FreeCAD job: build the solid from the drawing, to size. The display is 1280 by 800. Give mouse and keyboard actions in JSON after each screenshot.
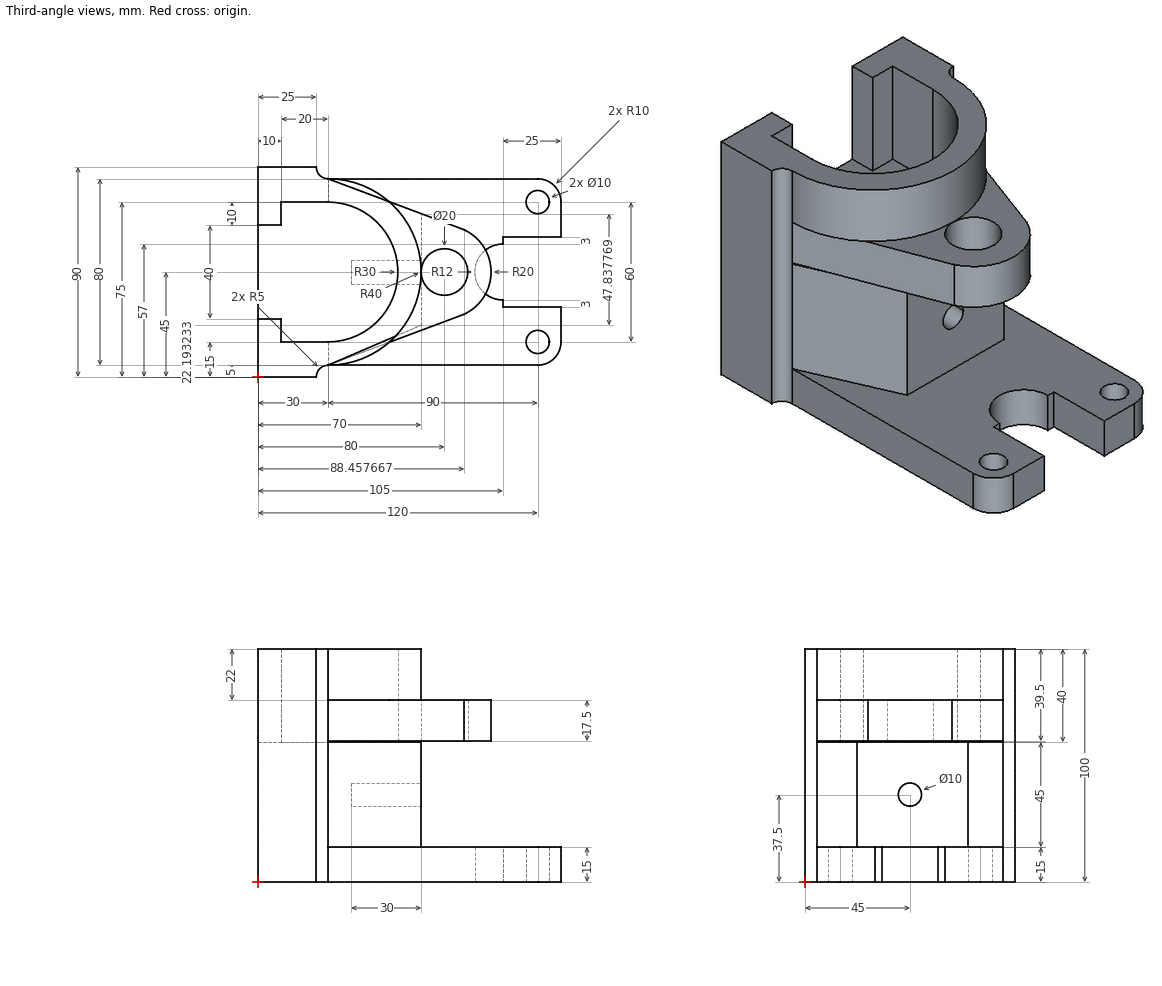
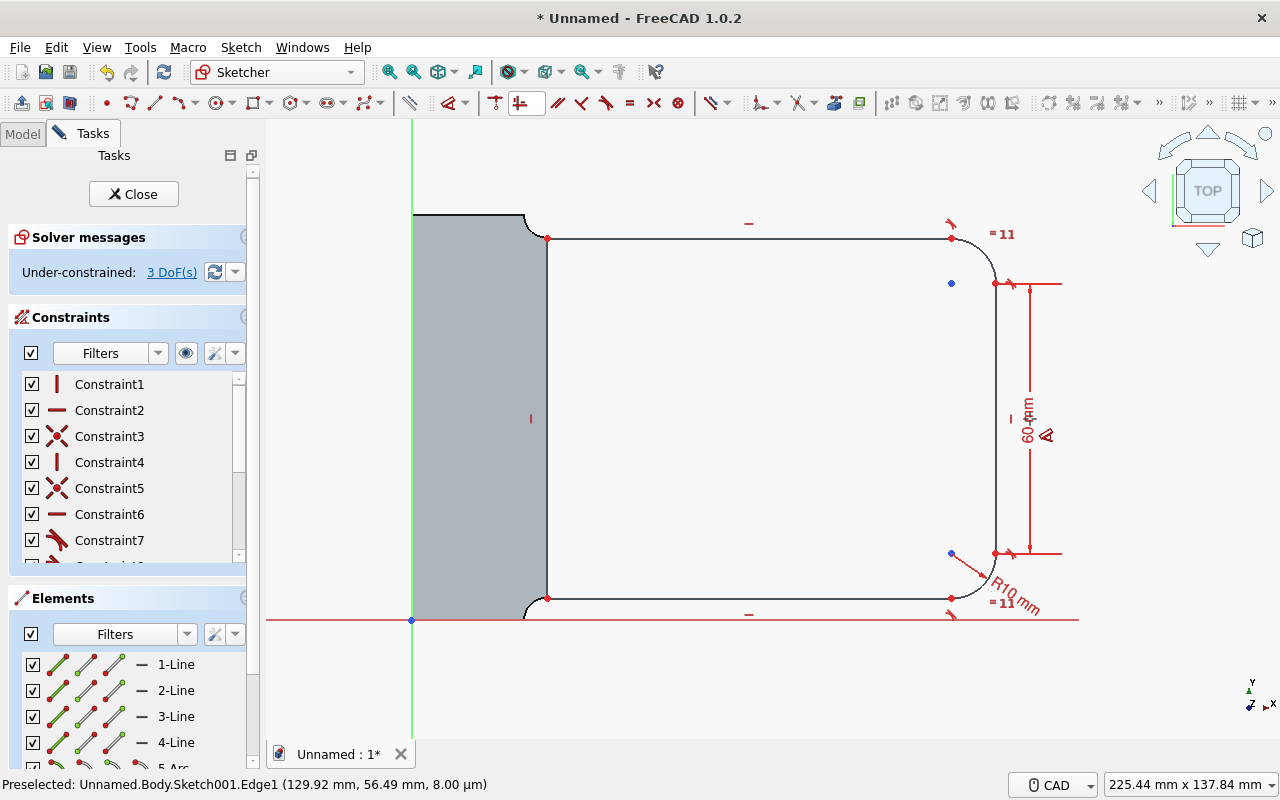
{"action": "left_click", "coordinate": [830, 599]}
{"action": "left_click", "coordinate": [749, 565]}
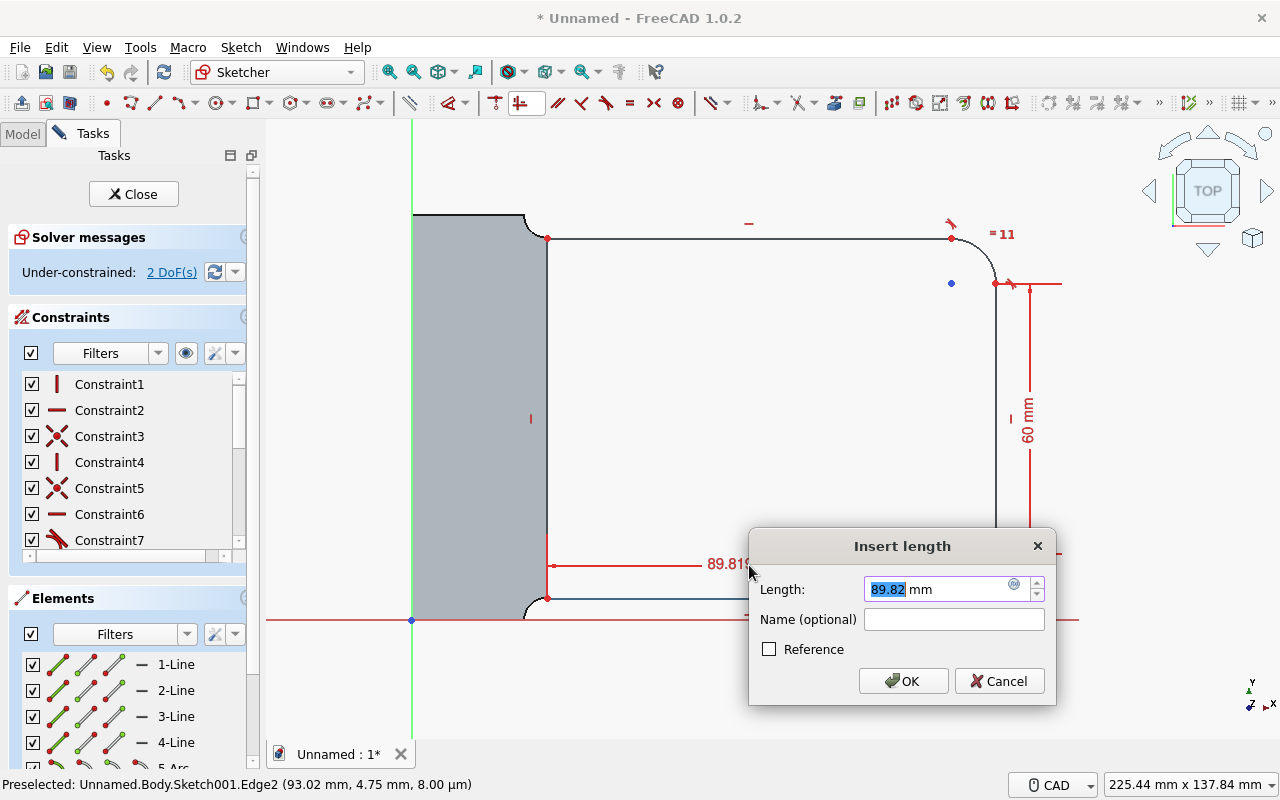
{"action": "type", "text": "90"}
{"action": "key", "text": "Return"}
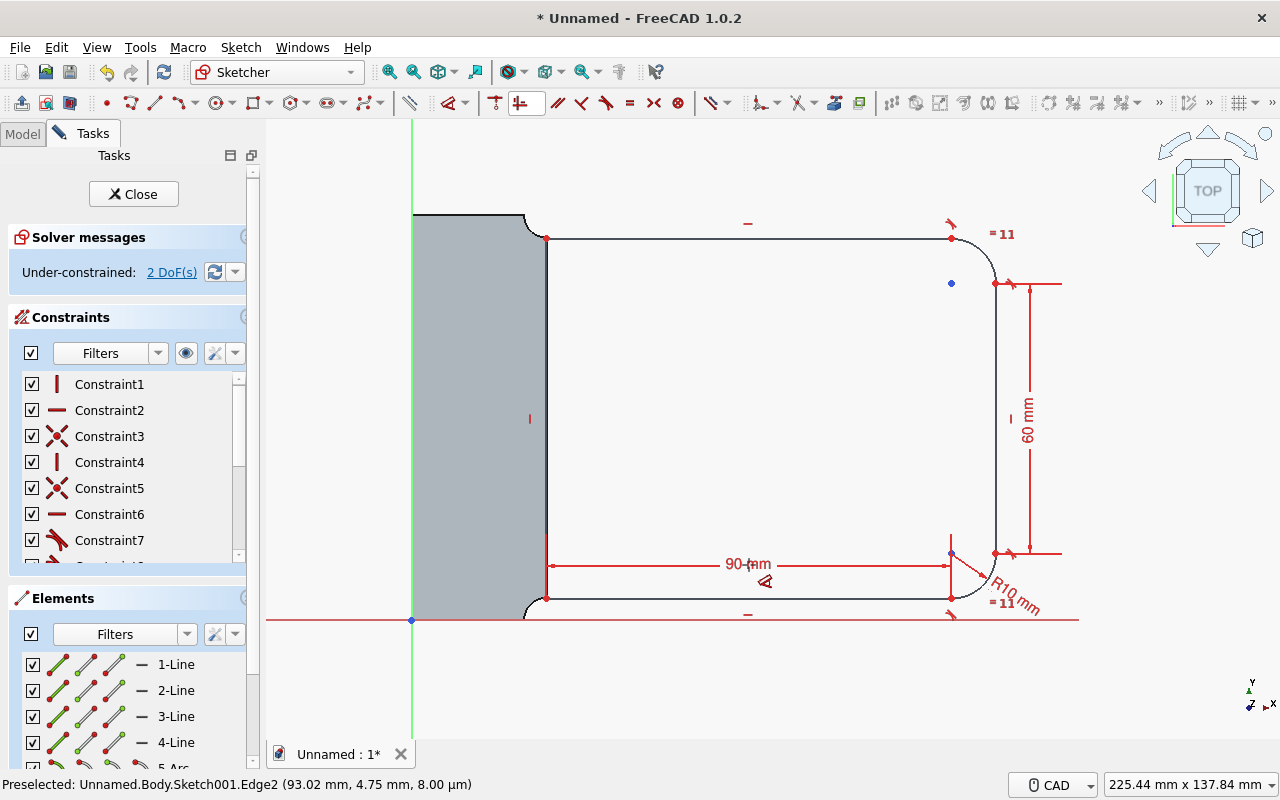
{"action": "scroll", "coordinate": [951, 599], "scroll_direction": "up", "scroll_amount": 3}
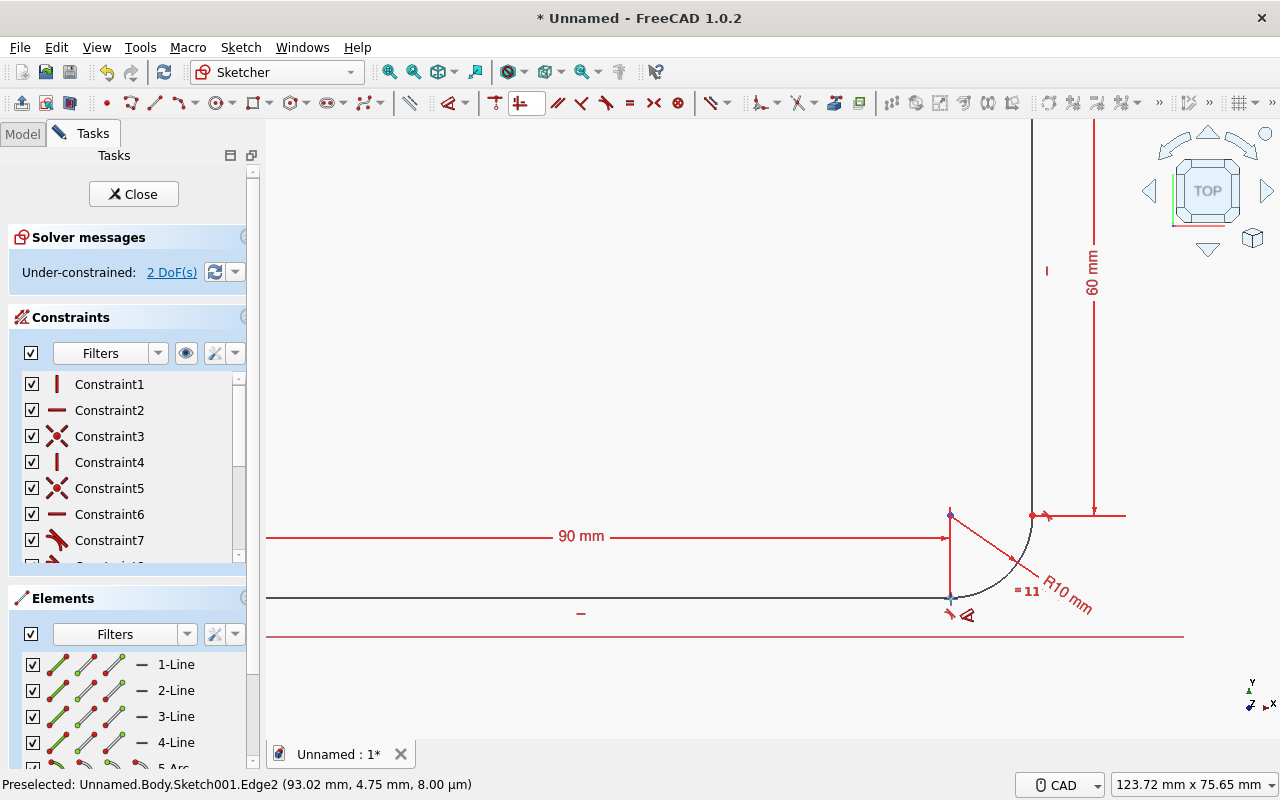
{"action": "left_click", "coordinate": [950, 598]}
{"action": "left_click", "coordinate": [984, 617]}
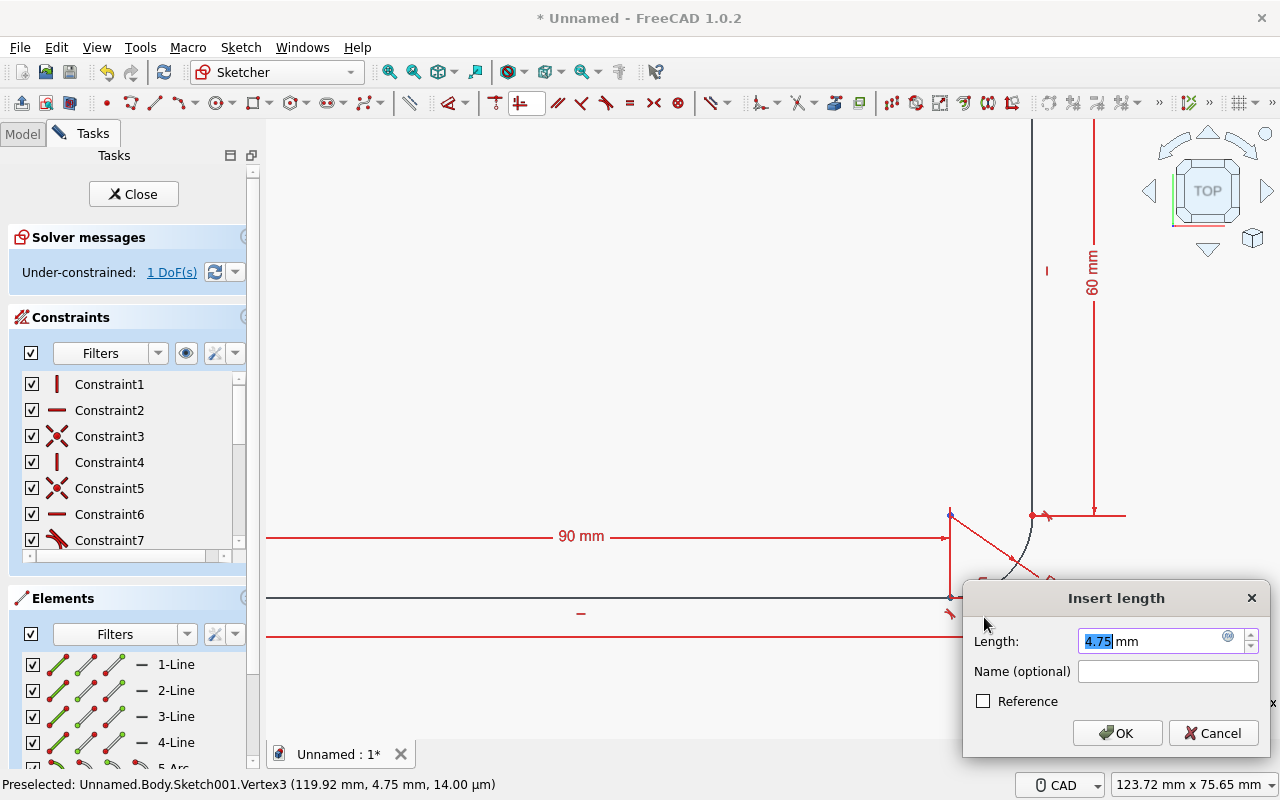
{"action": "type", "text": "5"}
{"action": "key", "text": "Return"}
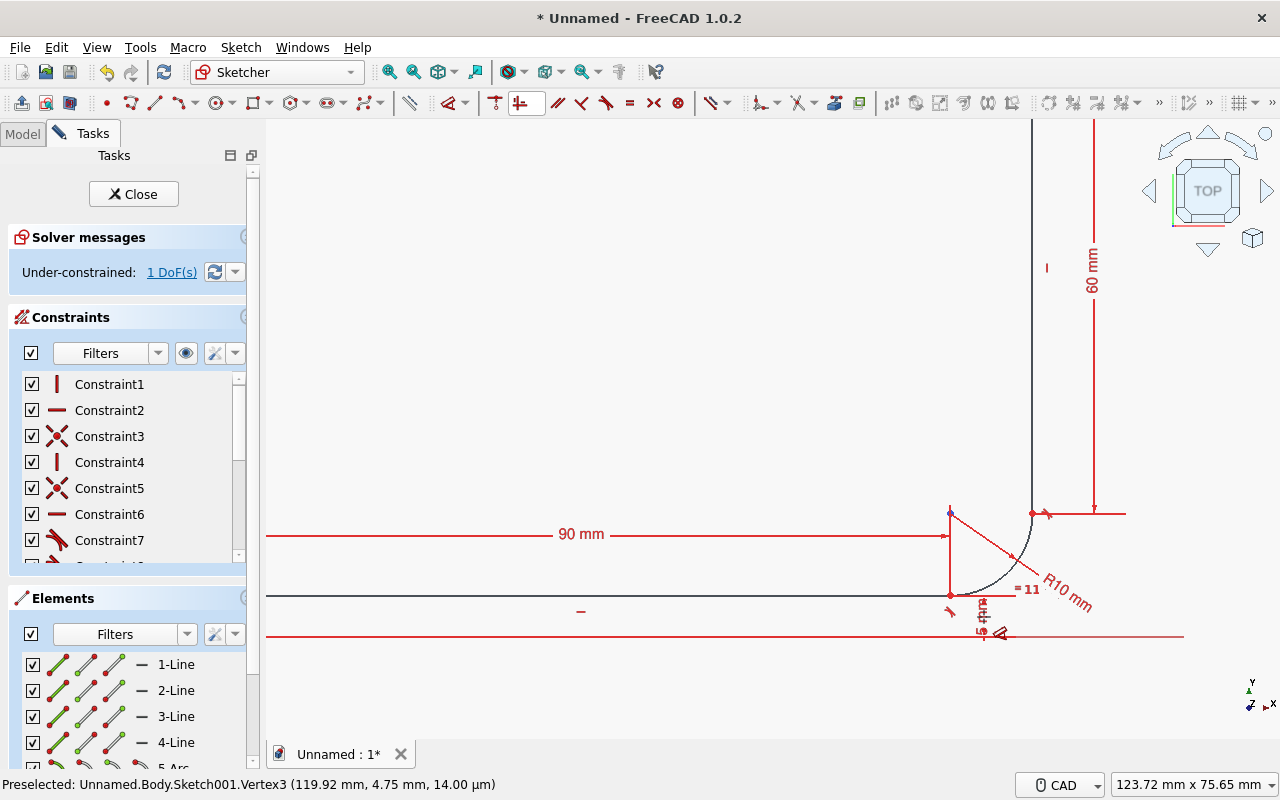
{"action": "scroll", "coordinate": [953, 600], "scroll_direction": "down", "scroll_amount": 3}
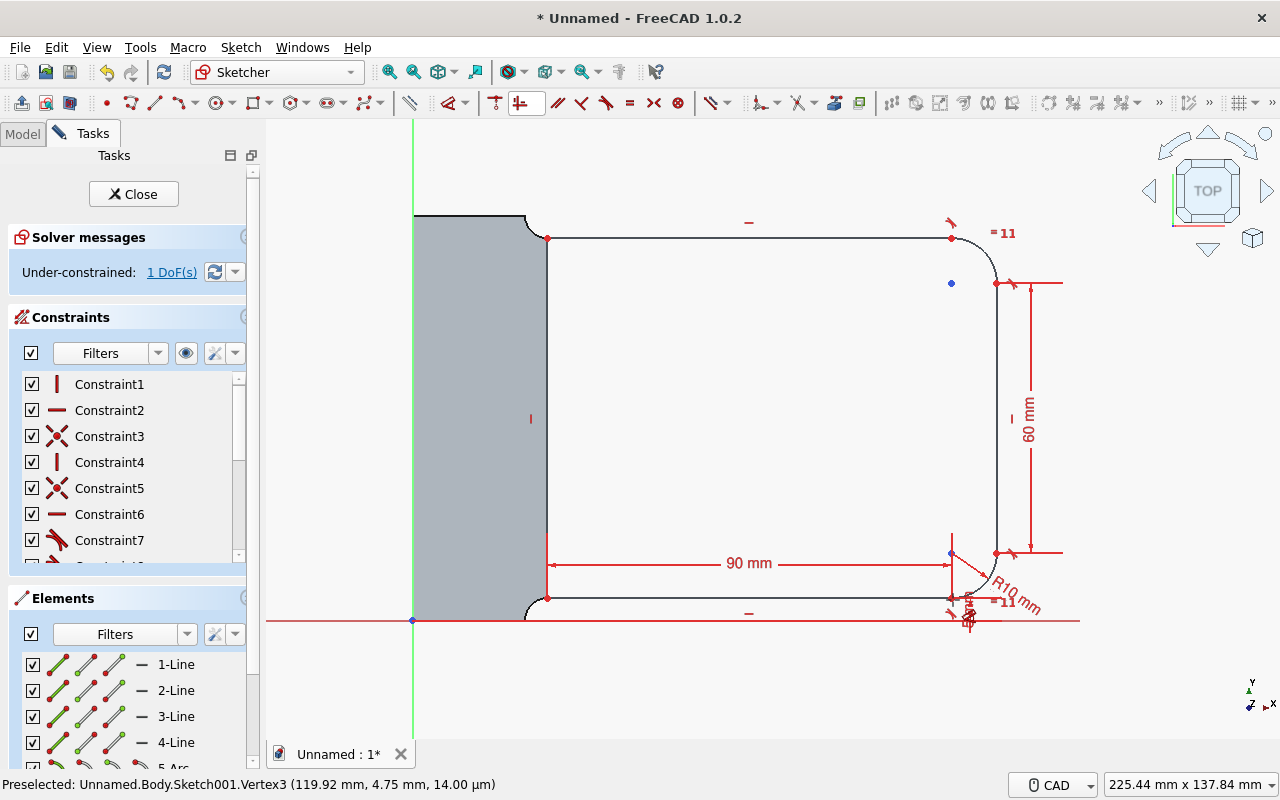
{"action": "left_click", "coordinate": [547, 598]}
{"action": "left_click", "coordinate": [480, 655]}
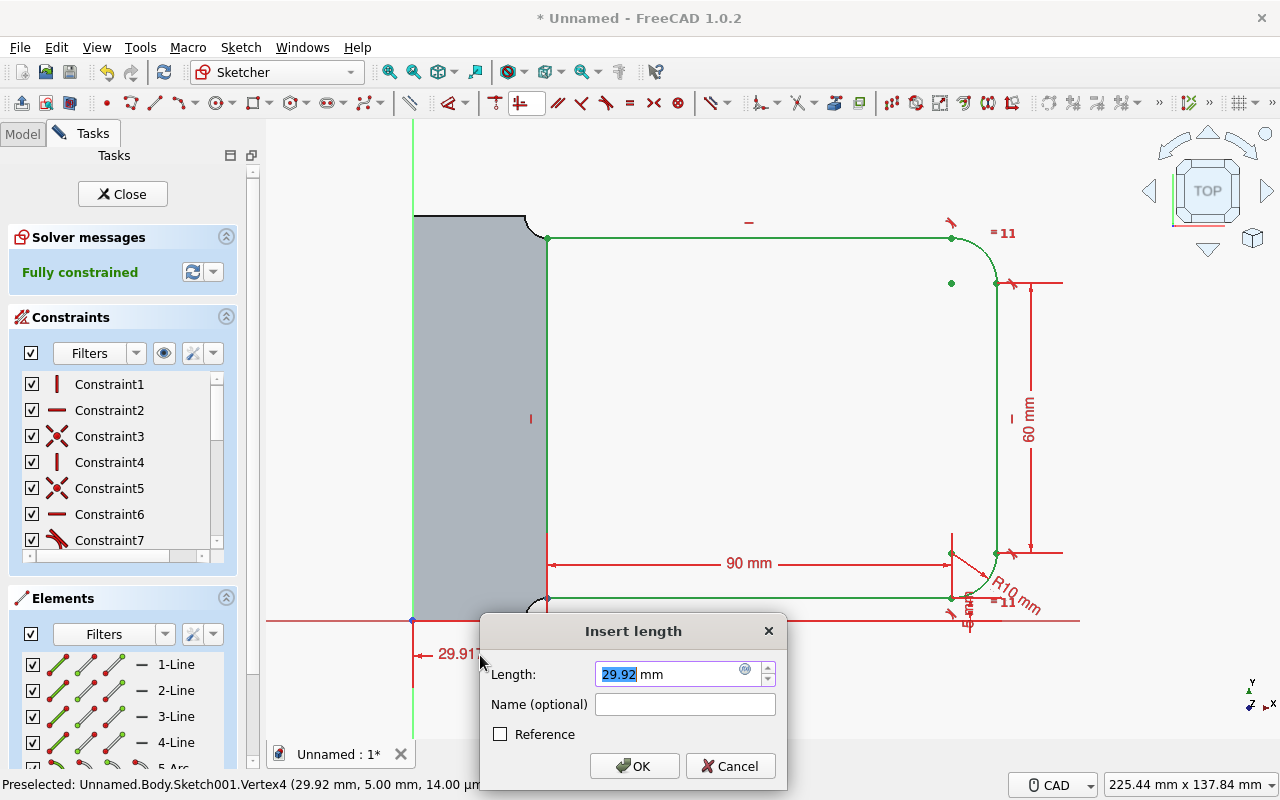
{"action": "type", "text": "30"}
{"action": "key", "text": "Return"}
{"action": "key", "text": "Escape"}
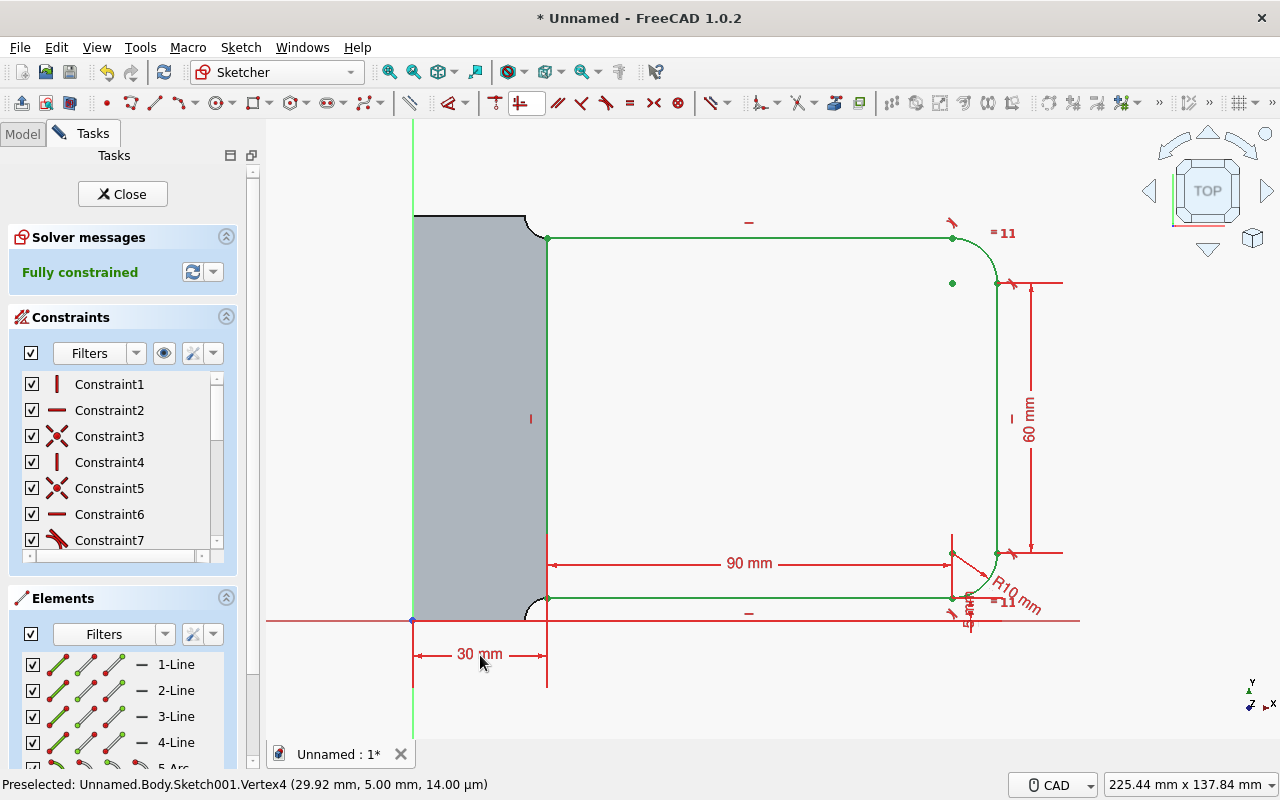
{"action": "left_click", "coordinate": [123, 194]}